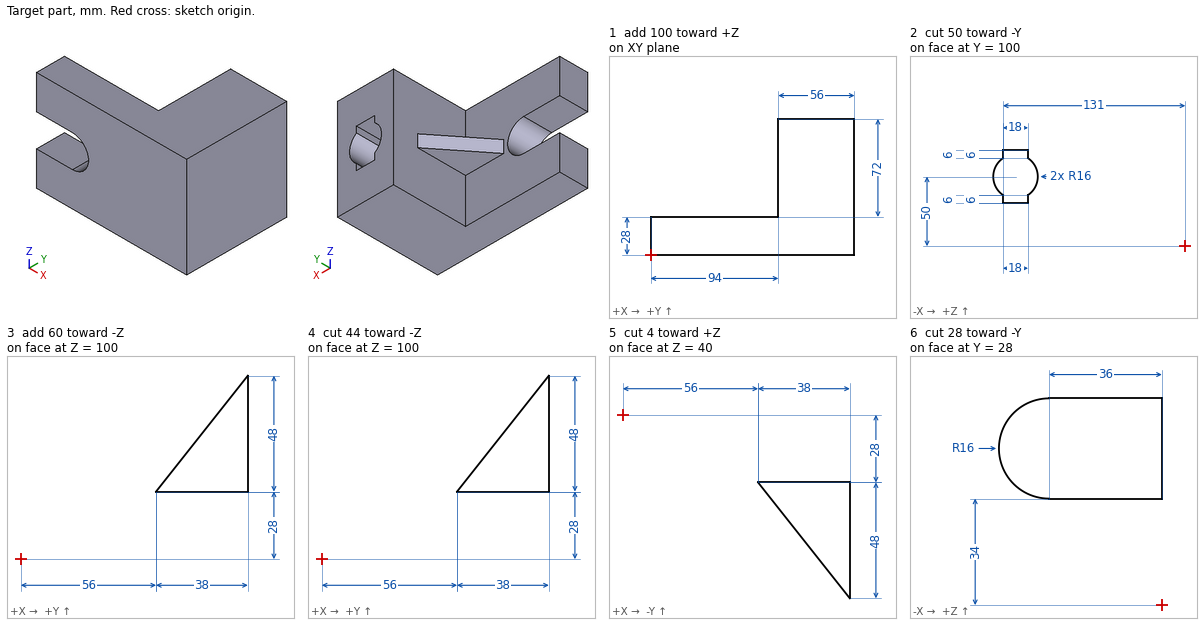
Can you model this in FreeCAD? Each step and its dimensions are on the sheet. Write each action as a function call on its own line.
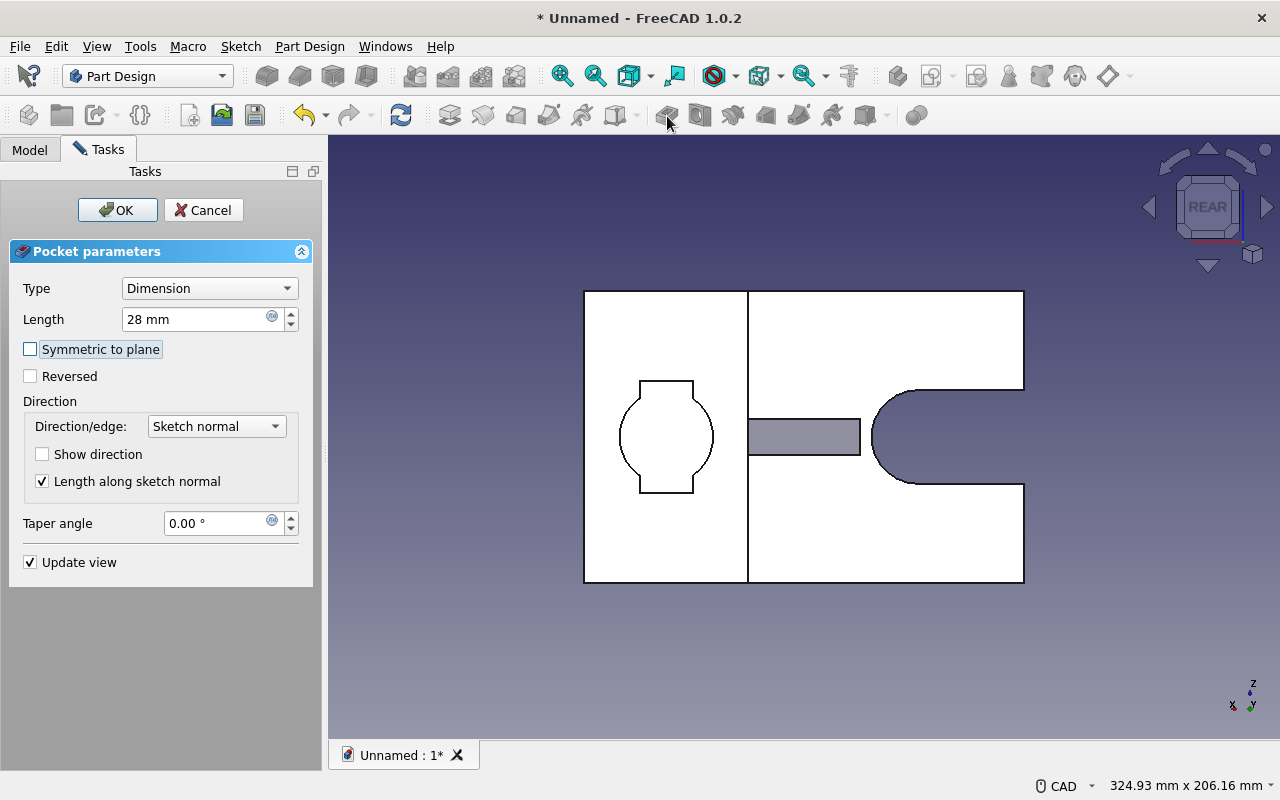
click(118, 210)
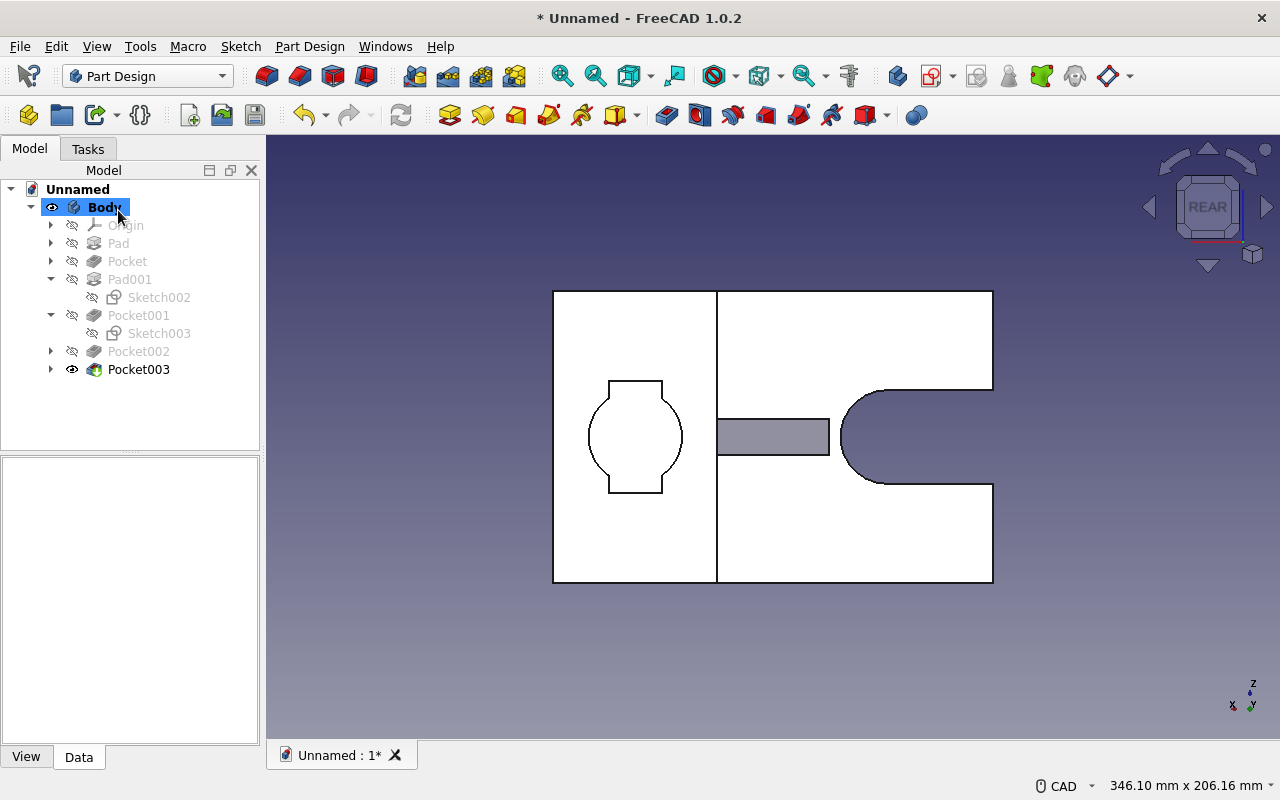
key(0)